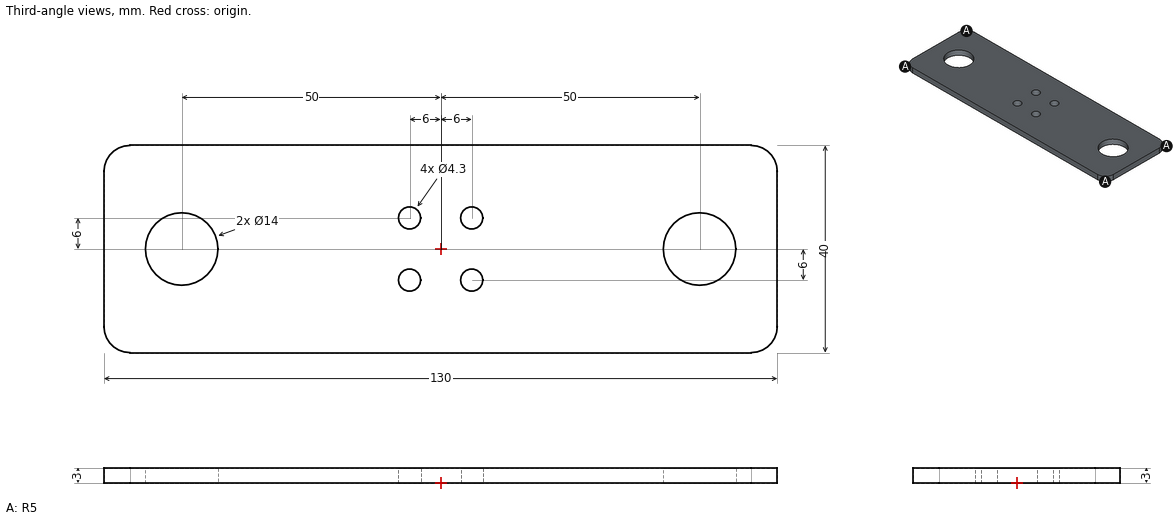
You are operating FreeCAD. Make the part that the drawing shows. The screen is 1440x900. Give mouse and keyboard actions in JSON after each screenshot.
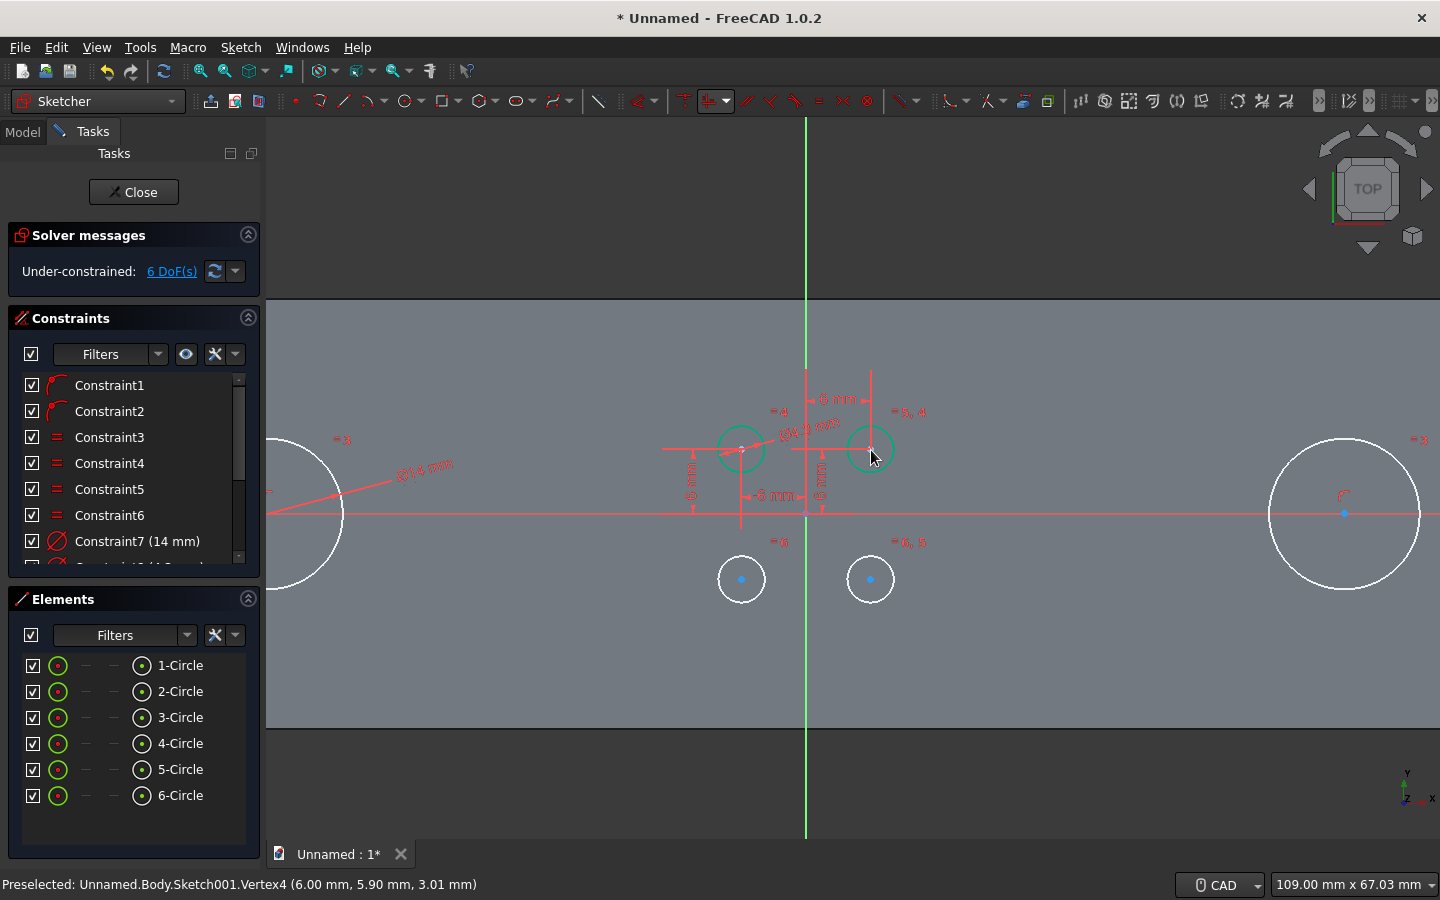
{"action": "left_click", "coordinate": [871, 579]}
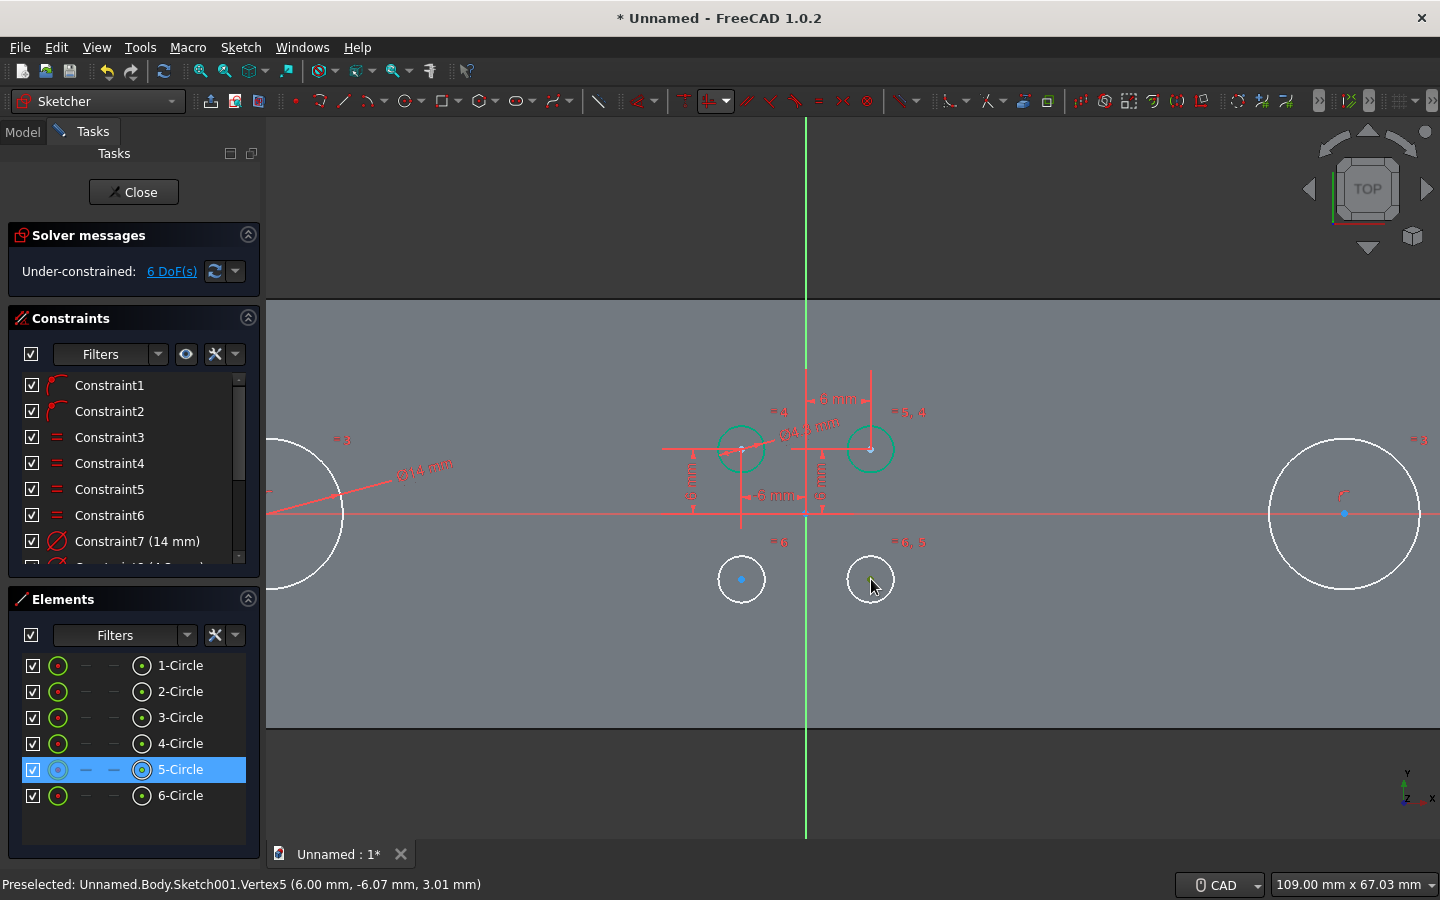
{"action": "left_click", "coordinate": [656, 102]}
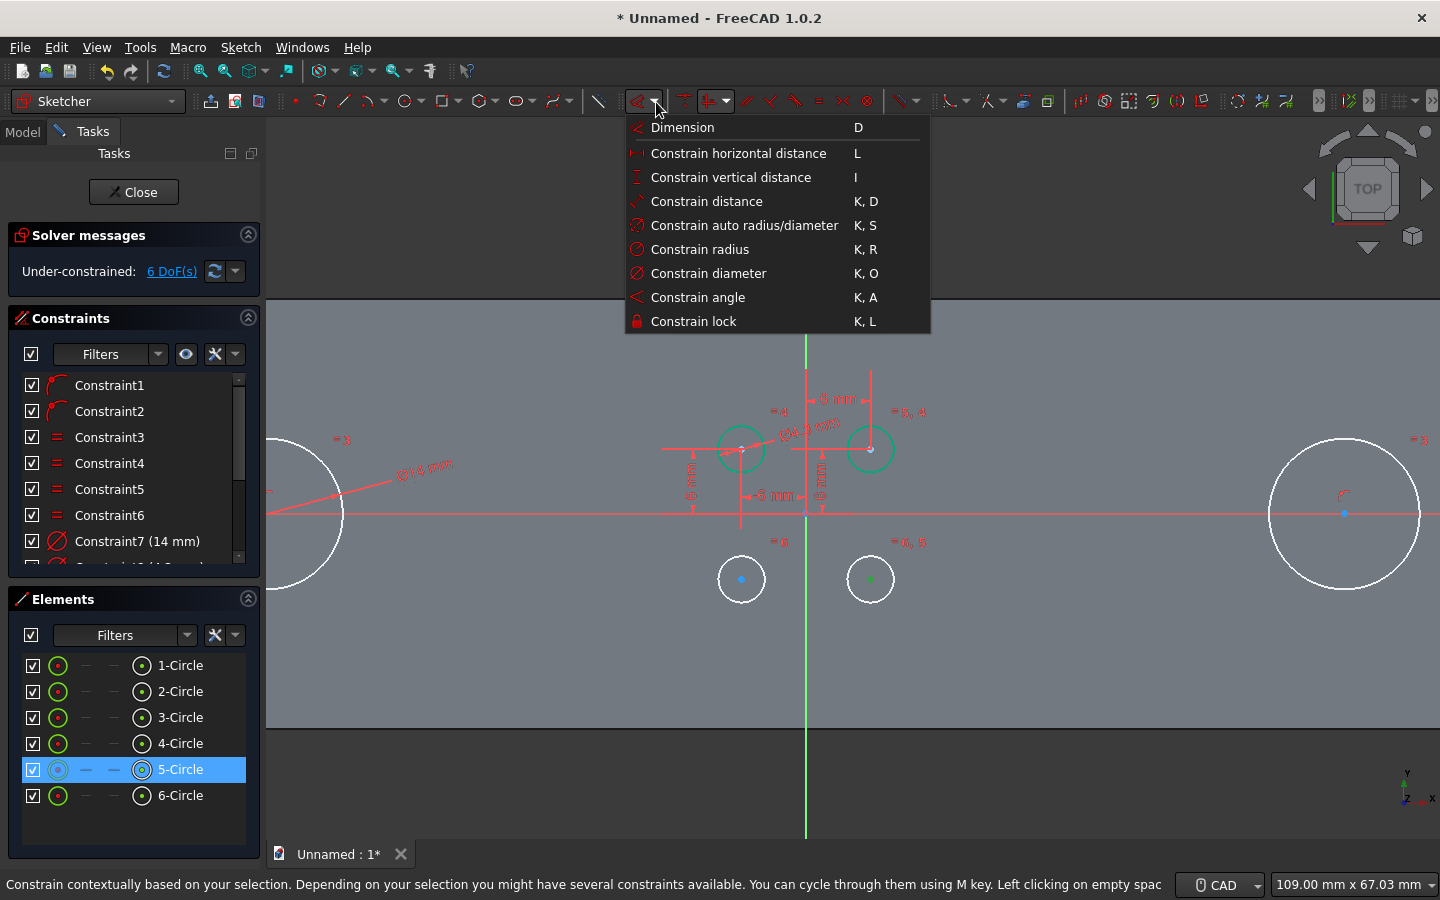
{"action": "left_click", "coordinate": [778, 153]}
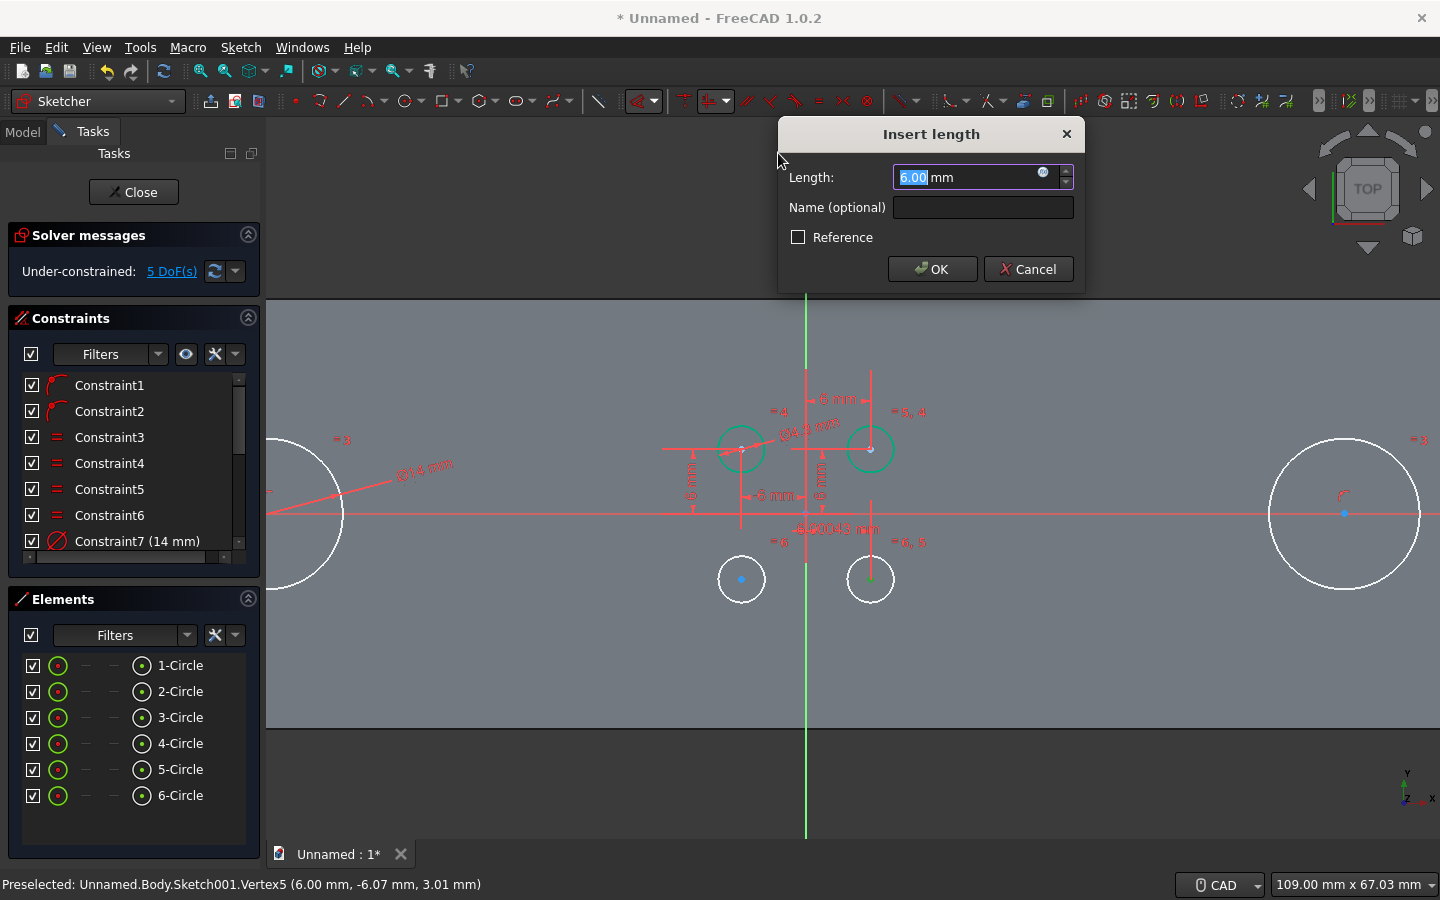
{"action": "type", "text": "6"}
{"action": "key", "text": "Return"}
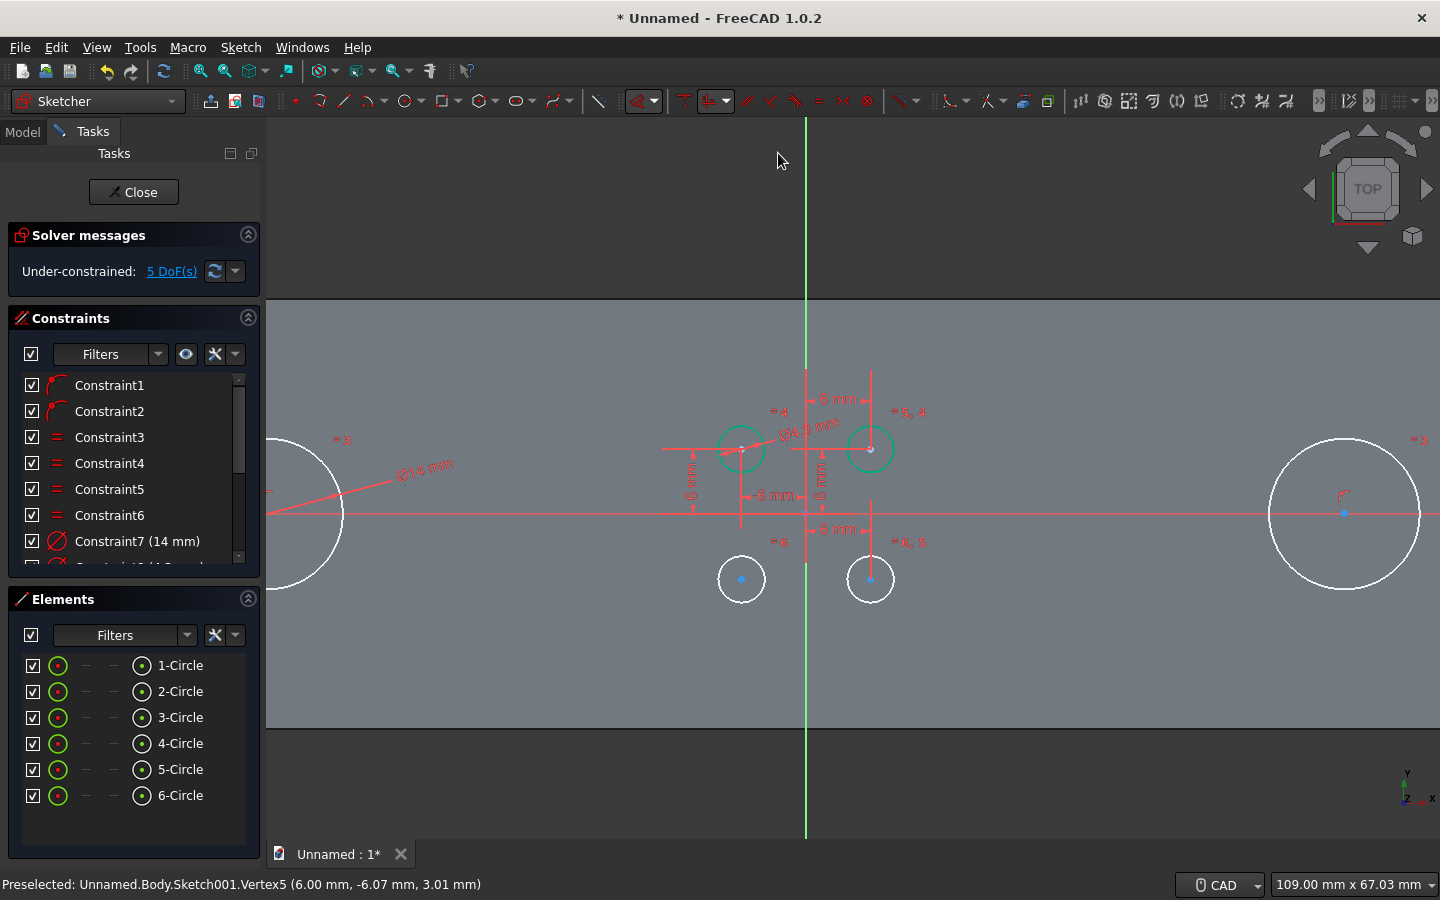
{"action": "left_click", "coordinate": [871, 579]}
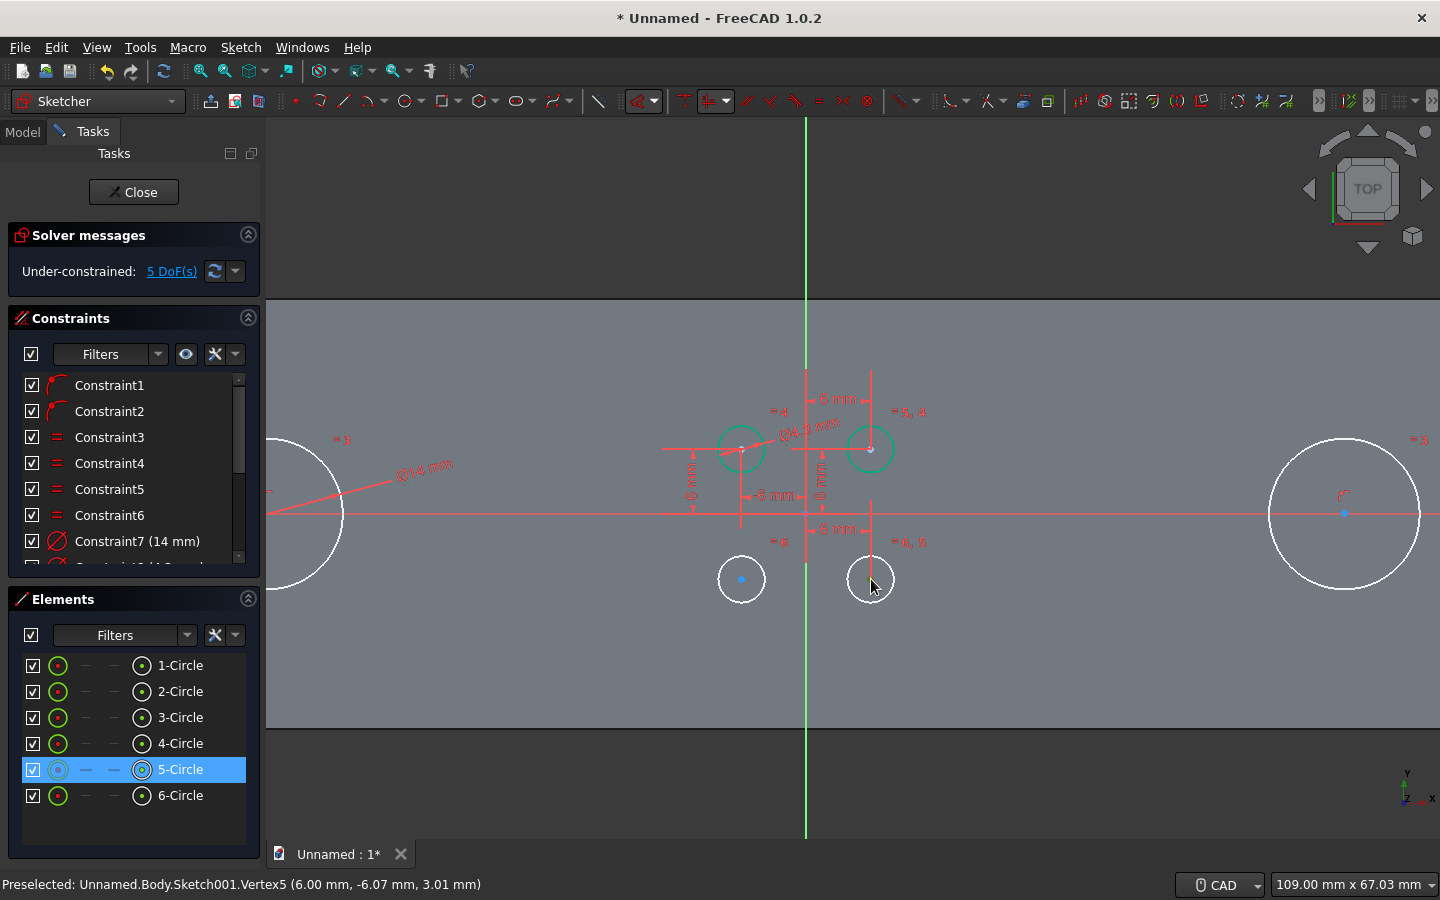
{"action": "left_click", "coordinate": [656, 102]}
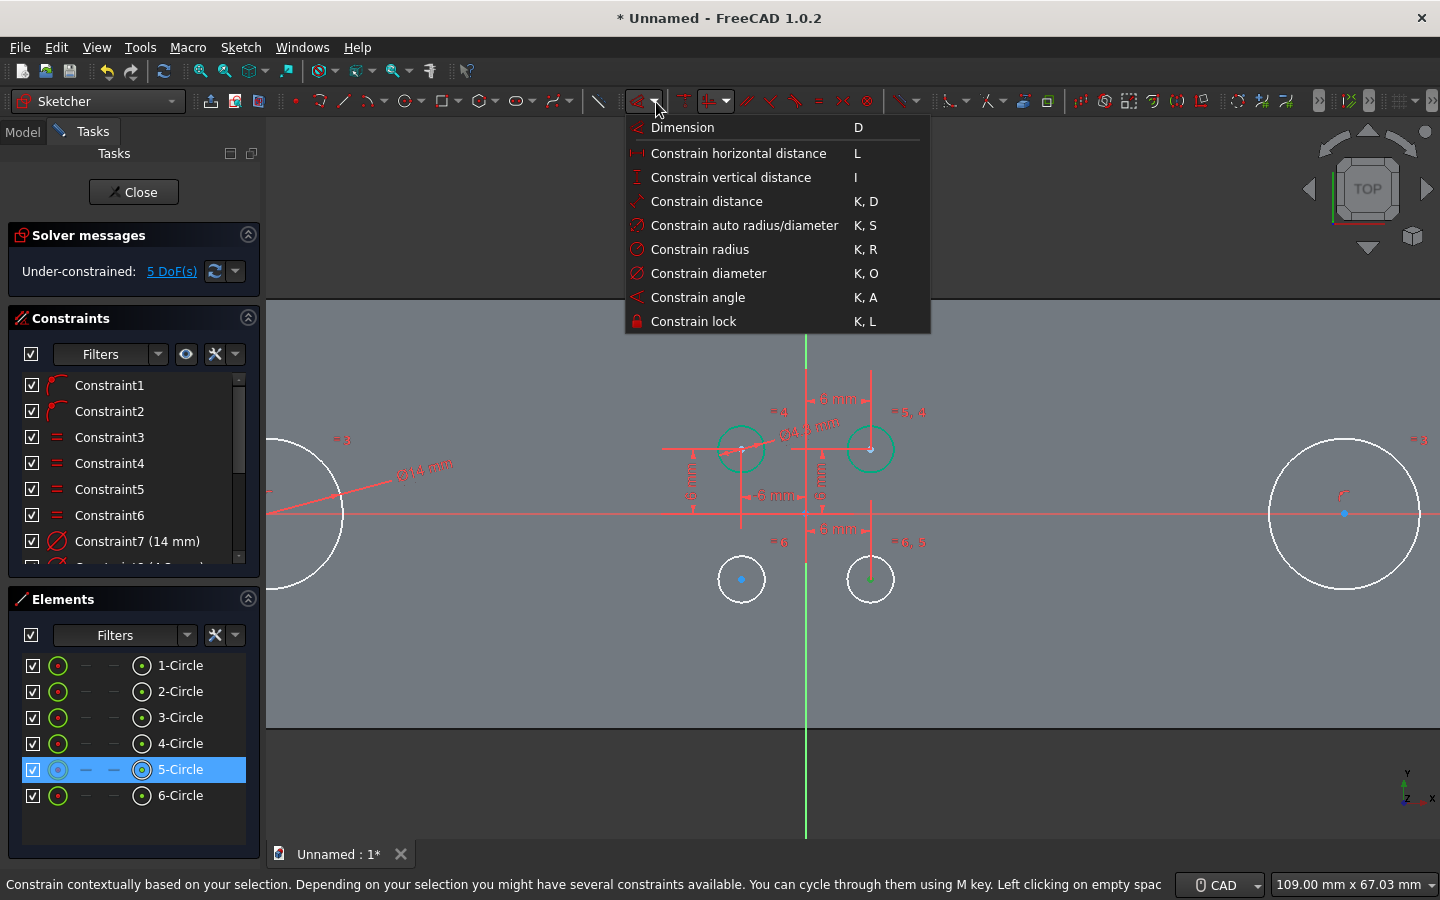
{"action": "left_click", "coordinate": [778, 177]}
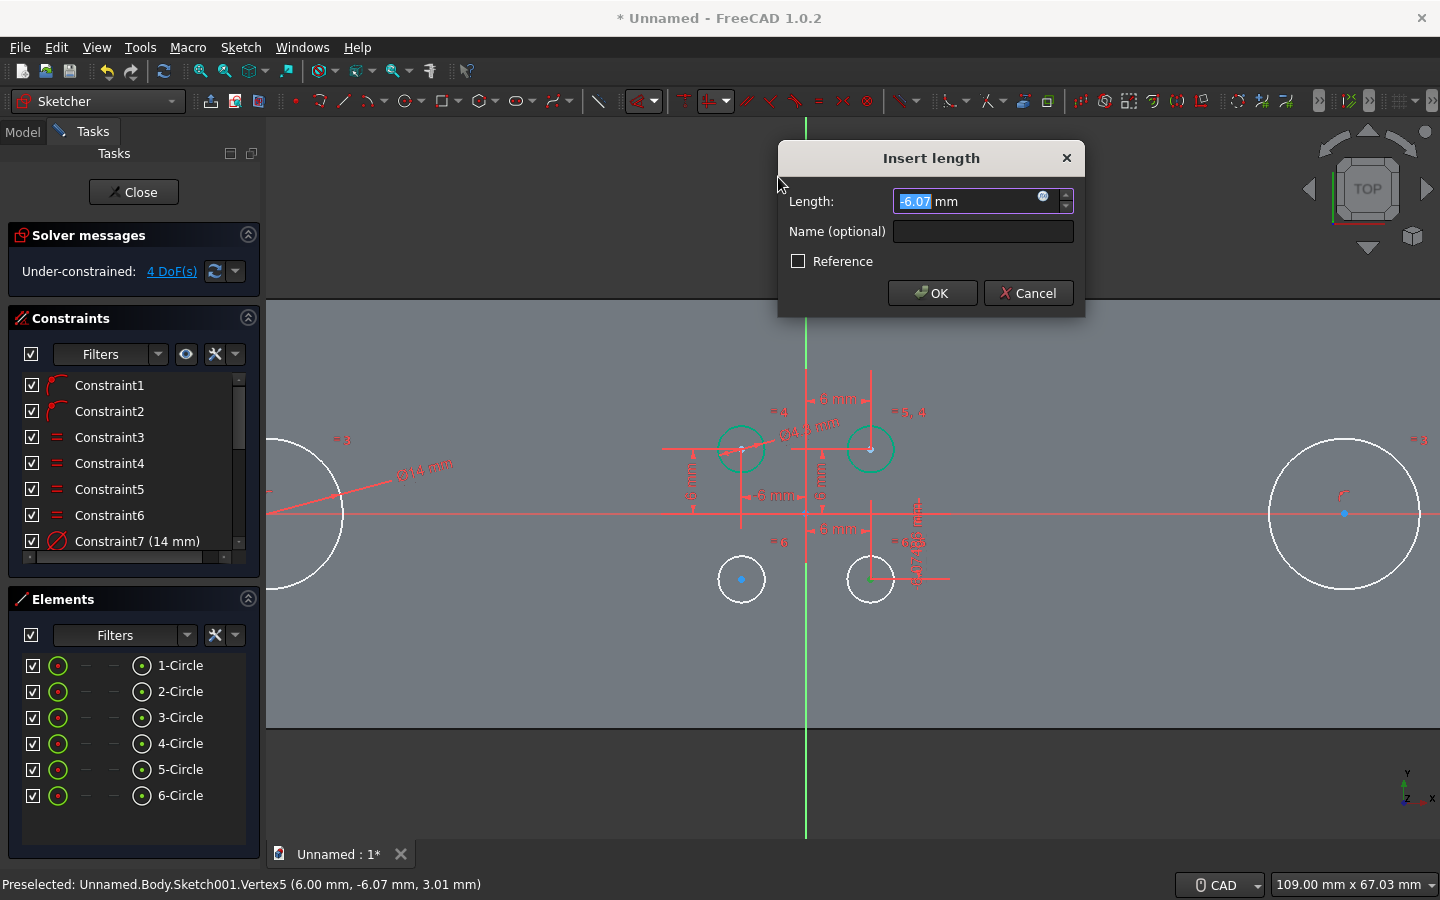
{"action": "type", "text": "-6"}
{"action": "key", "text": "Return"}